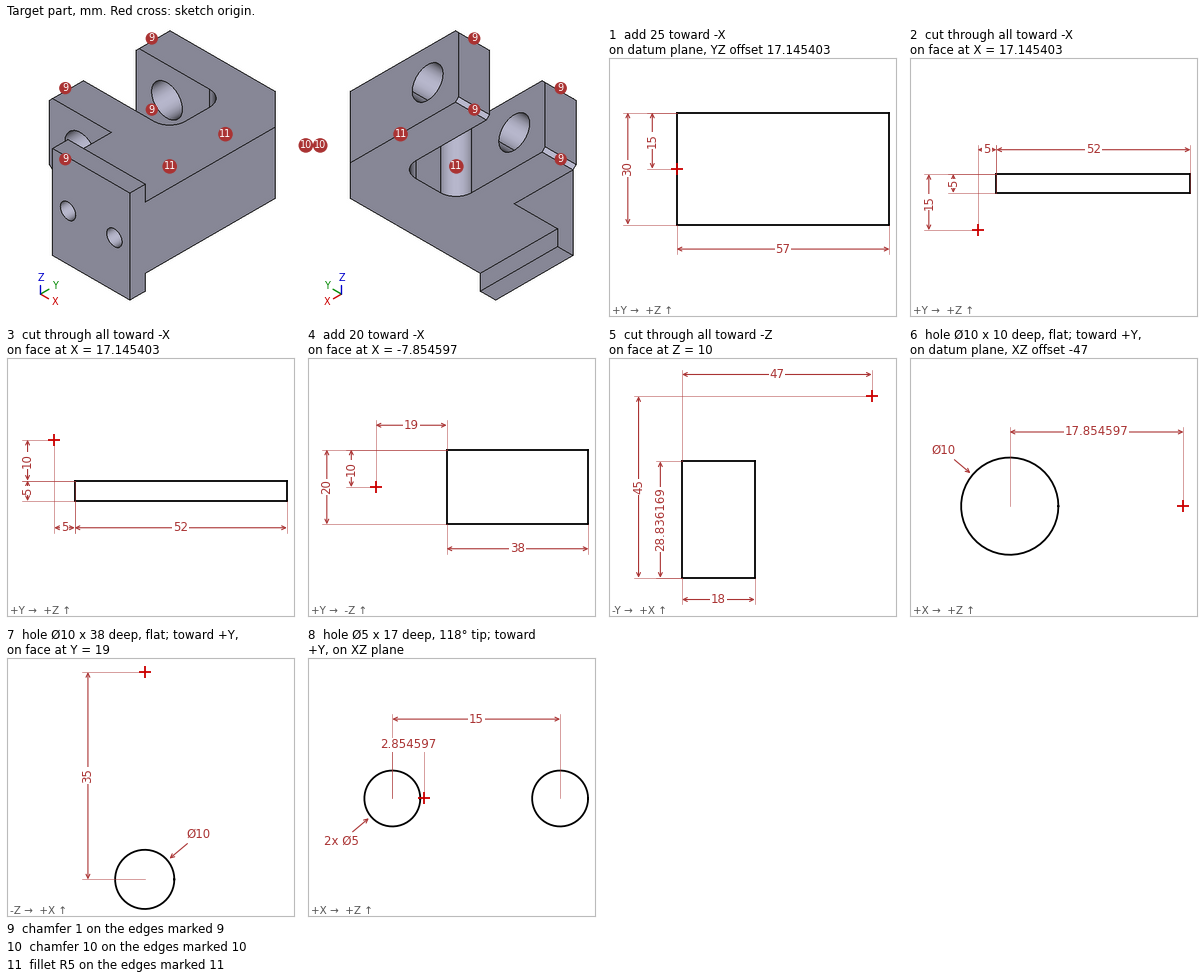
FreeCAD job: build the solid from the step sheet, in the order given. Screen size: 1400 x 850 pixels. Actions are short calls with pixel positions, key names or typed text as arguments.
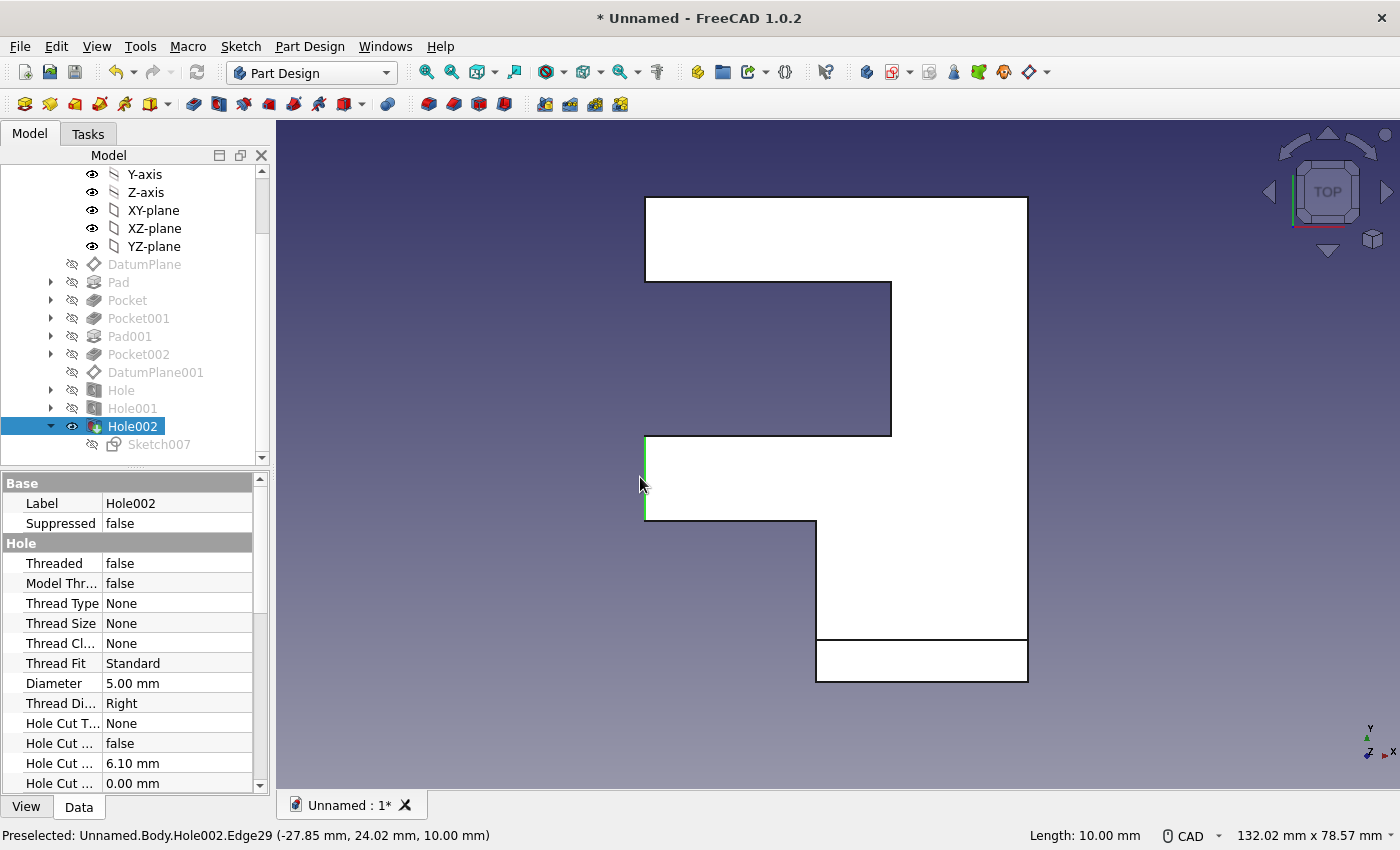
click(645, 239, ctrl)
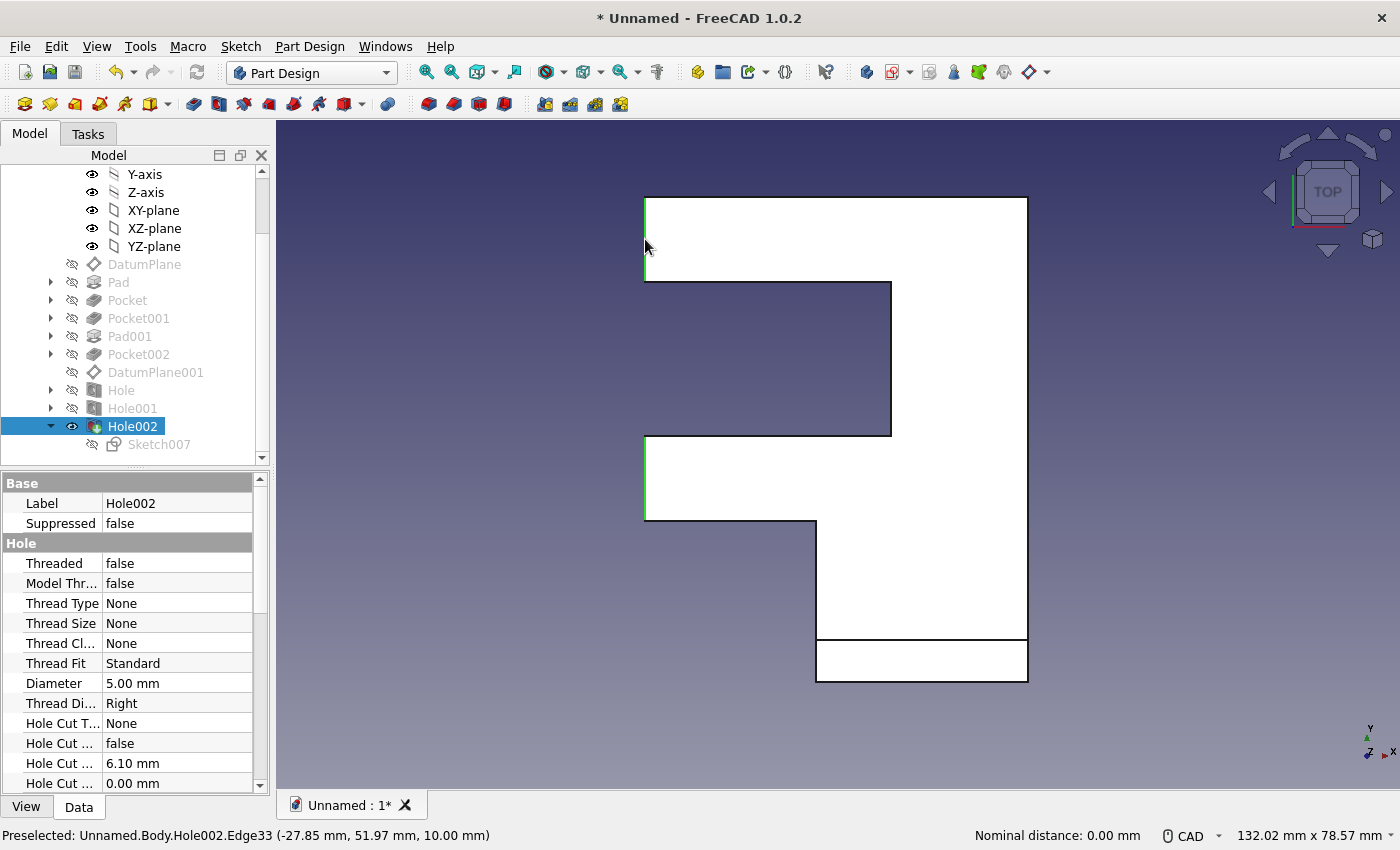
key(0)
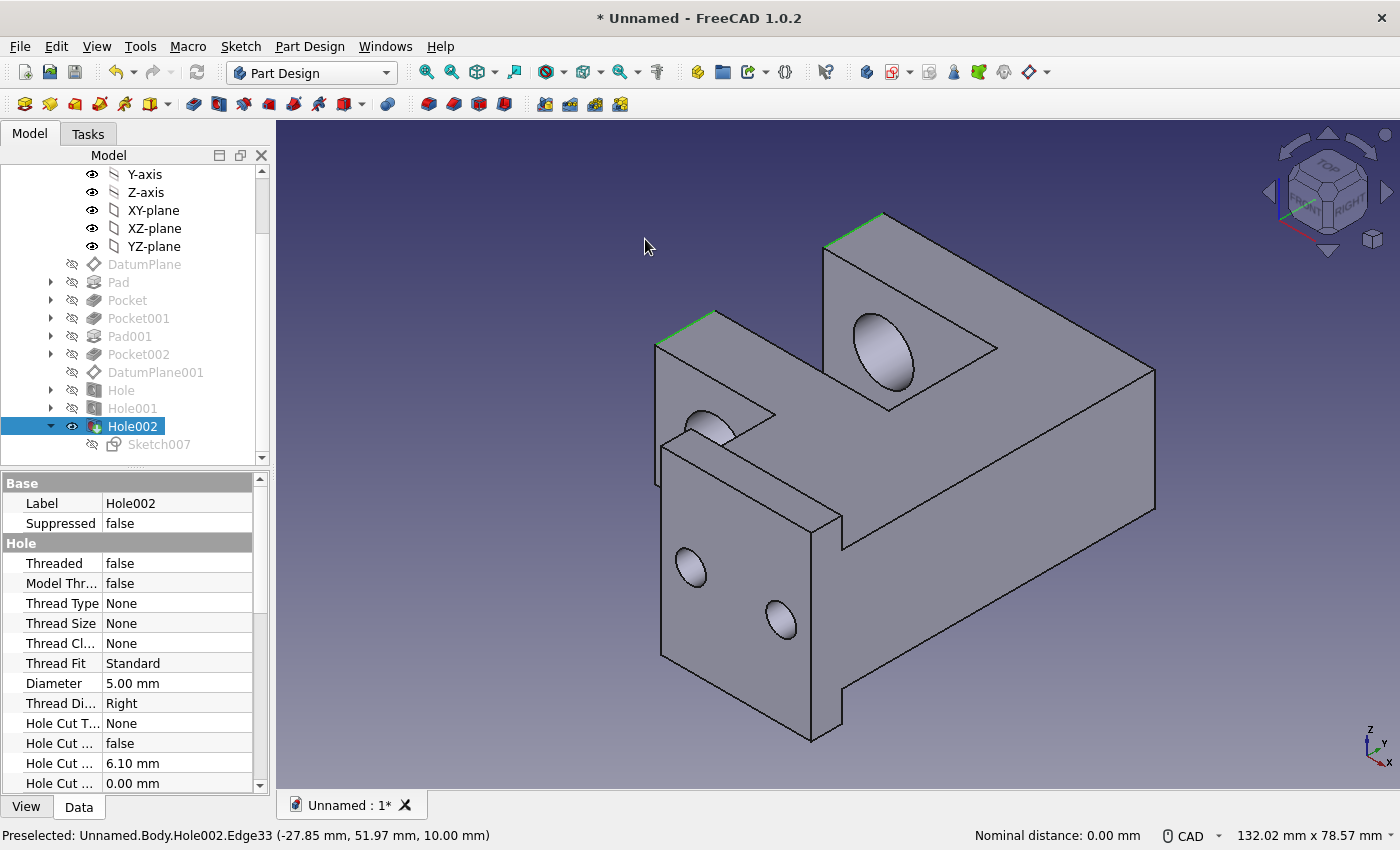
key(1)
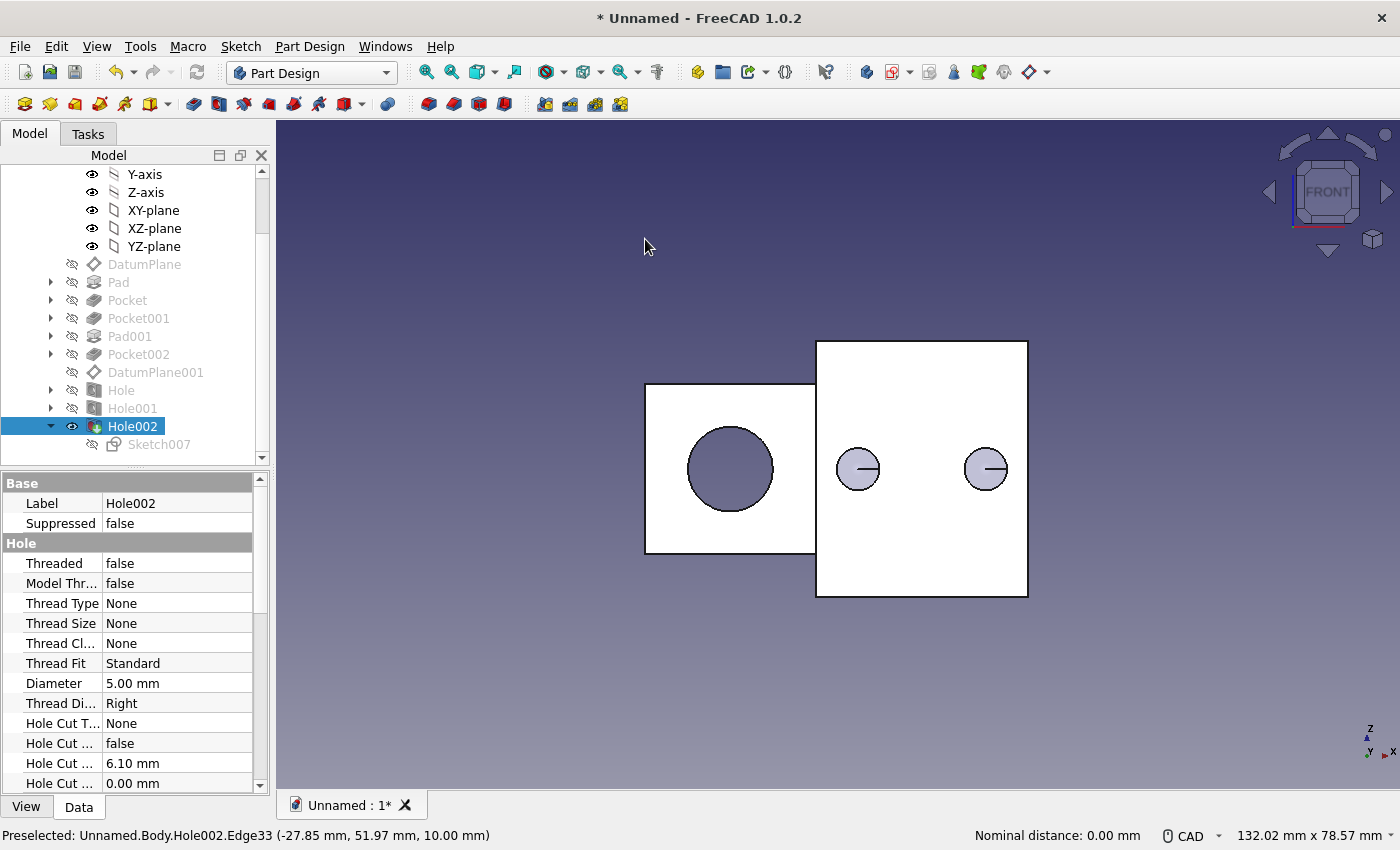
click(427, 72)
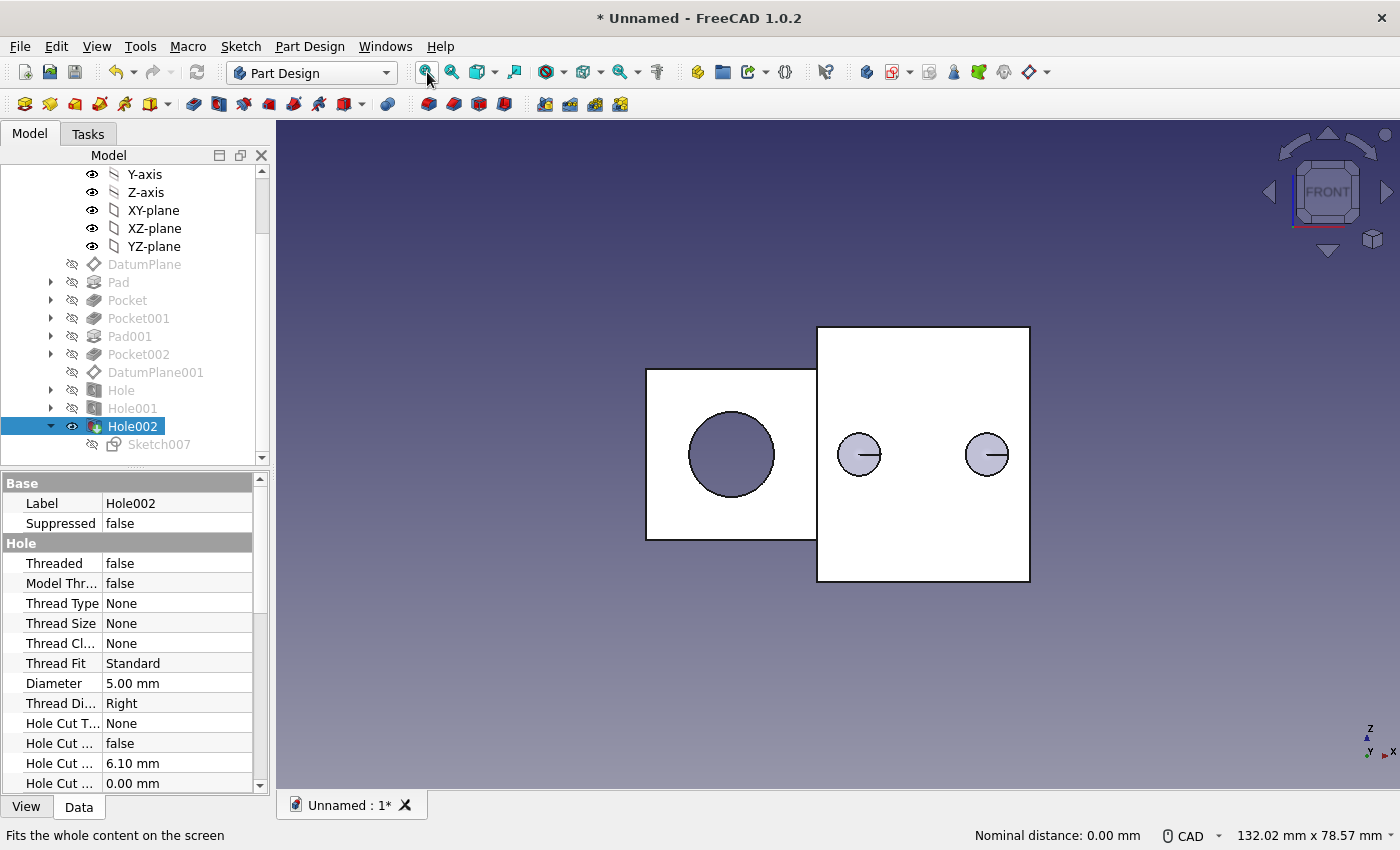
key(3)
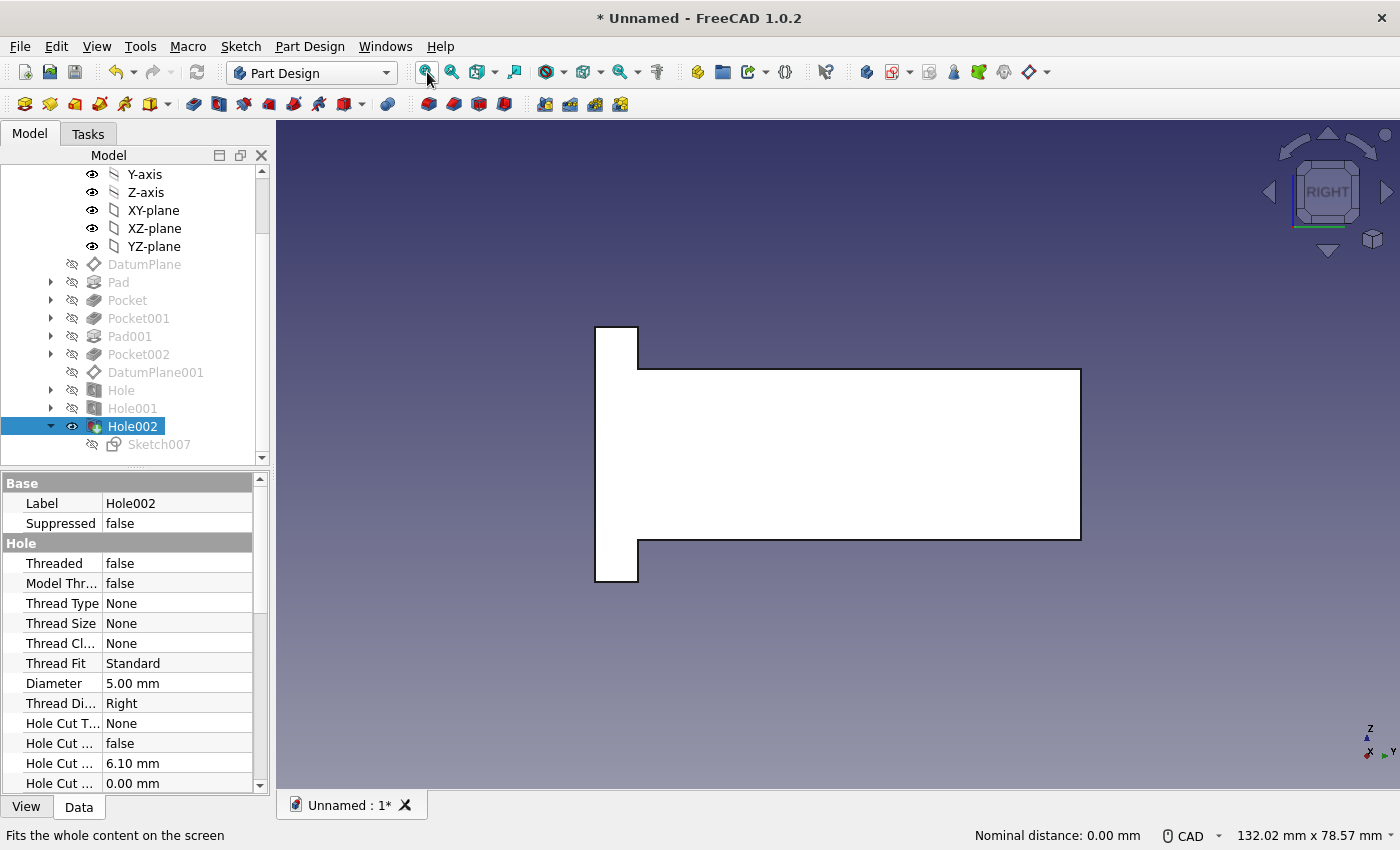
click(427, 72)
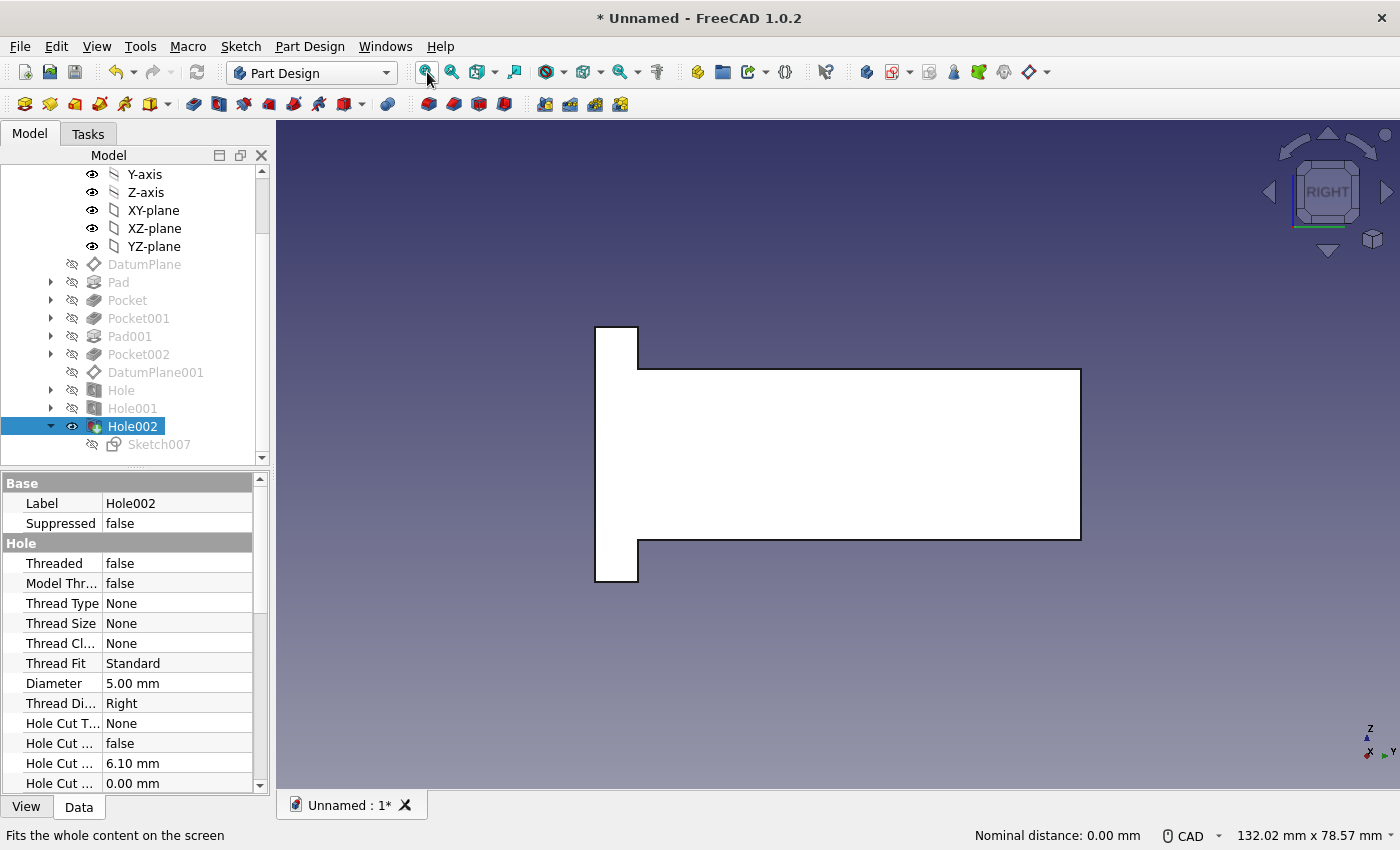
key(5)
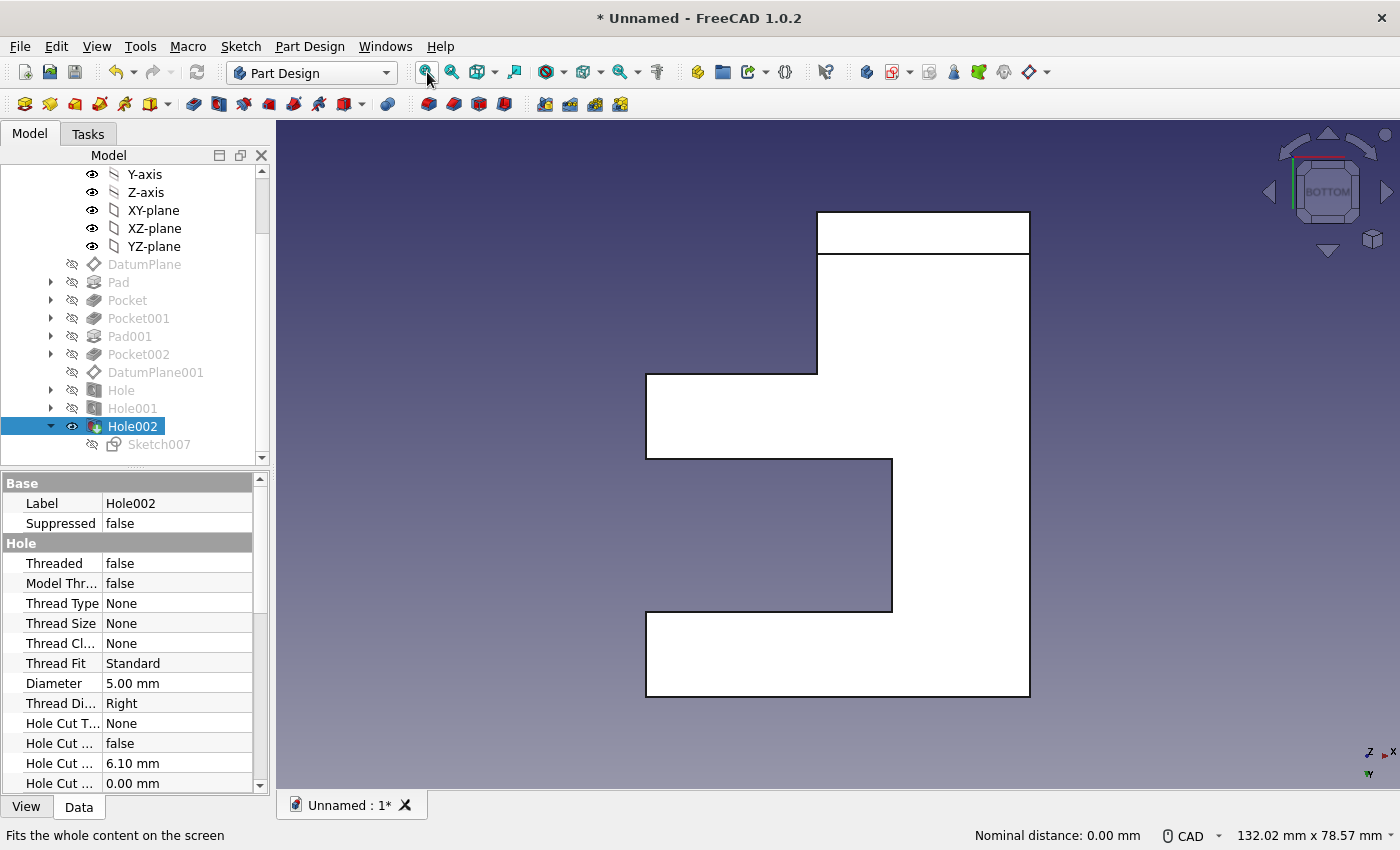
click(646, 654, ctrl)